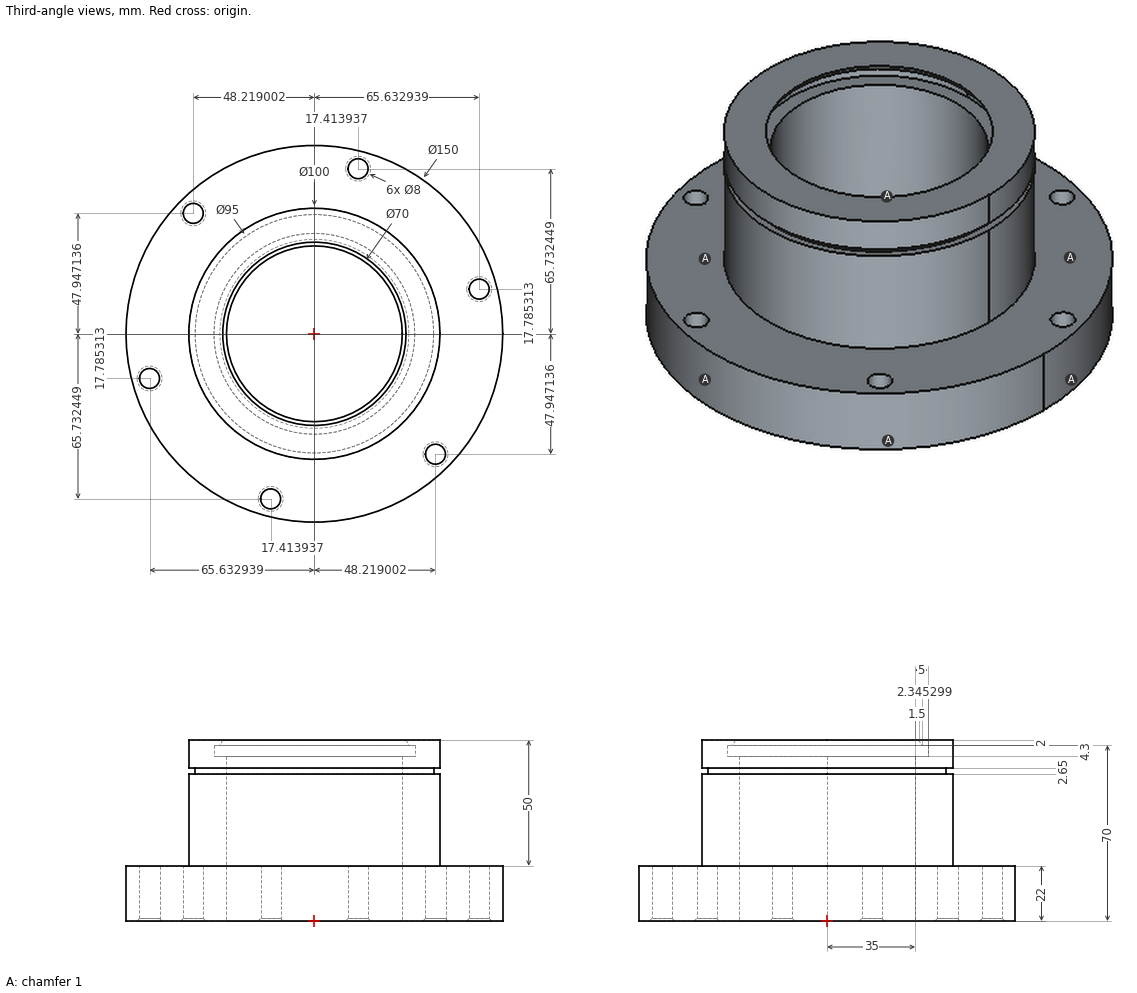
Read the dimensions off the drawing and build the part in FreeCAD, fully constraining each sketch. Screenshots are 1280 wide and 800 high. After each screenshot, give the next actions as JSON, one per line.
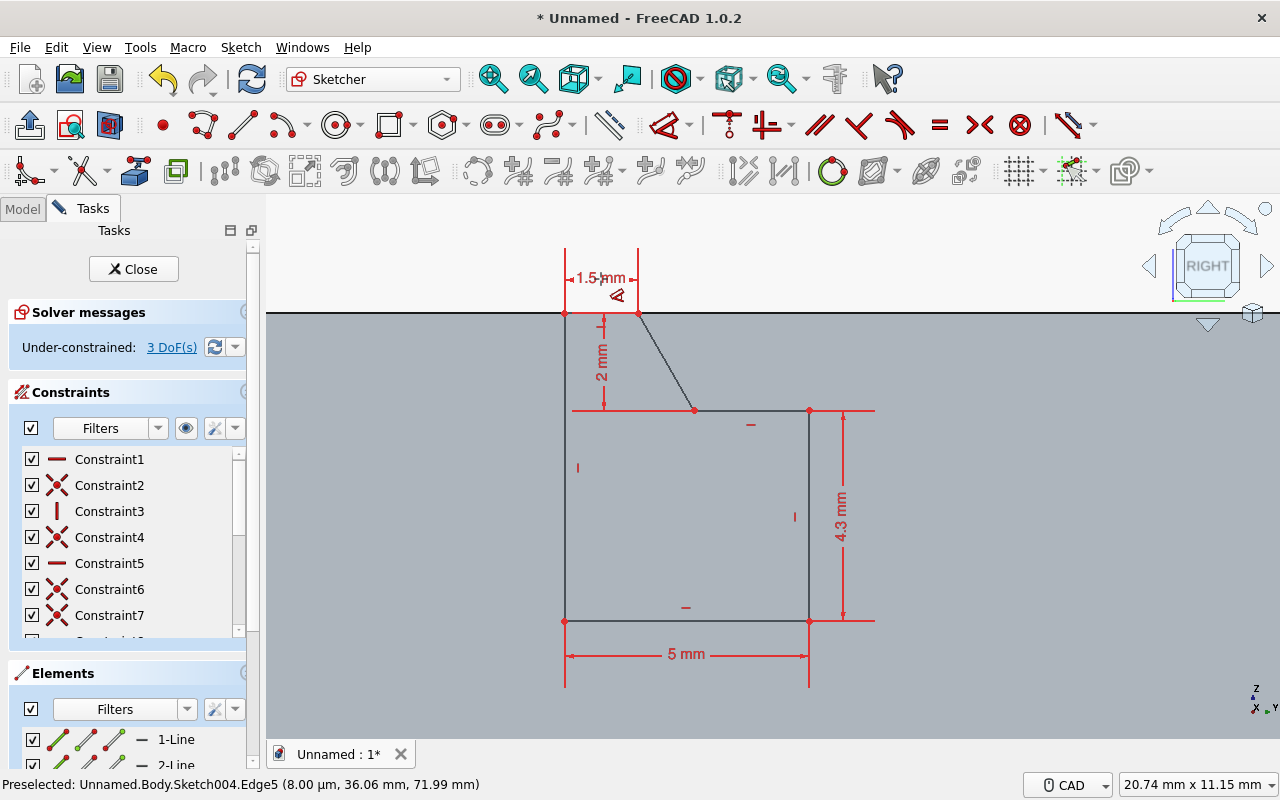
{"action": "left_click", "coordinate": [565, 621]}
{"action": "left_click", "coordinate": [429, 587]}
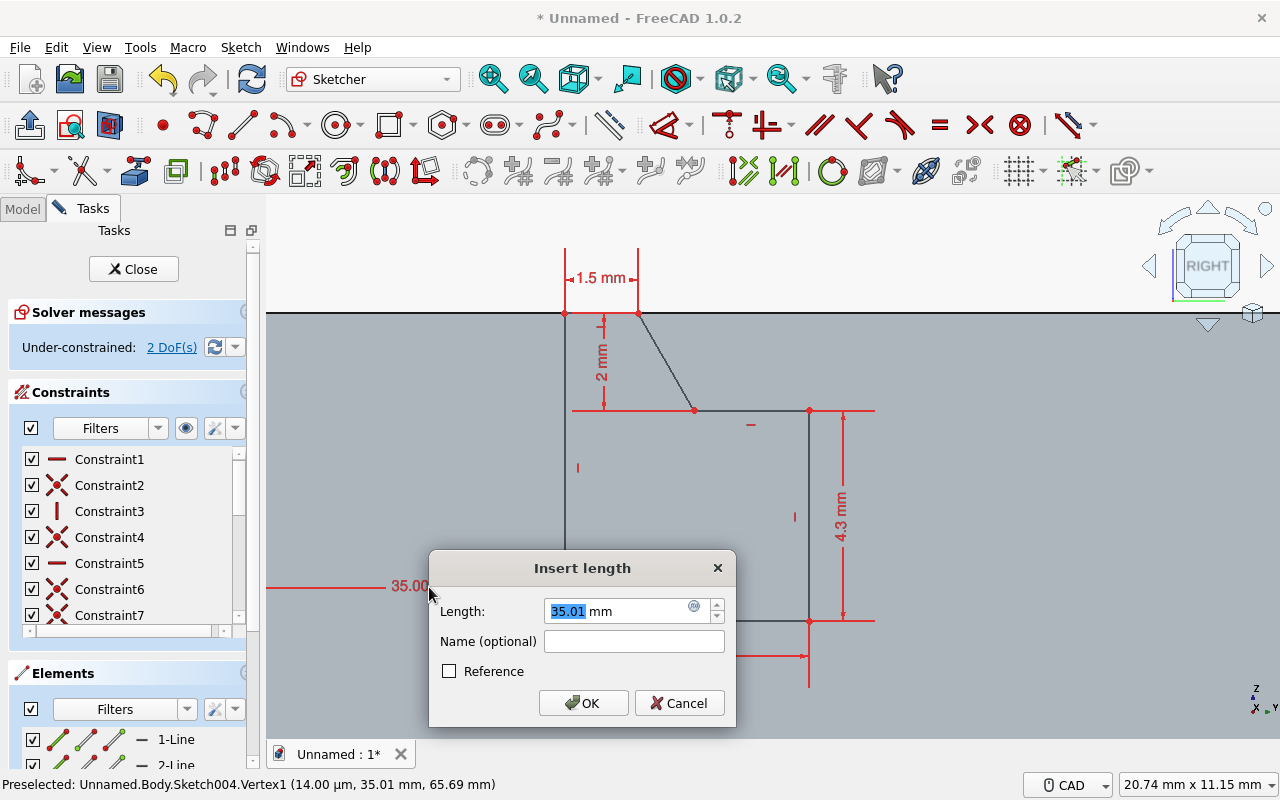
{"action": "type", "text": "35"}
{"action": "key", "text": "Return"}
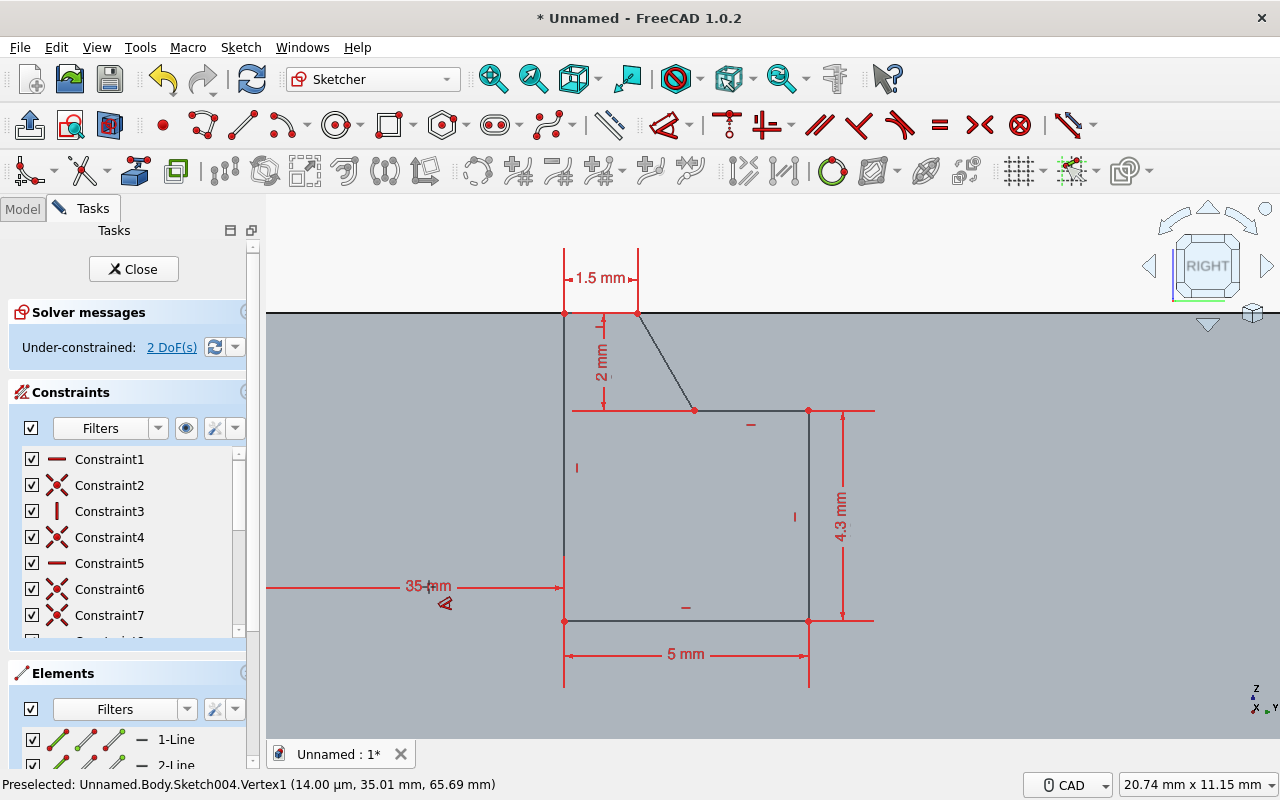
{"action": "left_click", "coordinate": [809, 411]}
{"action": "left_click", "coordinate": [843, 561]}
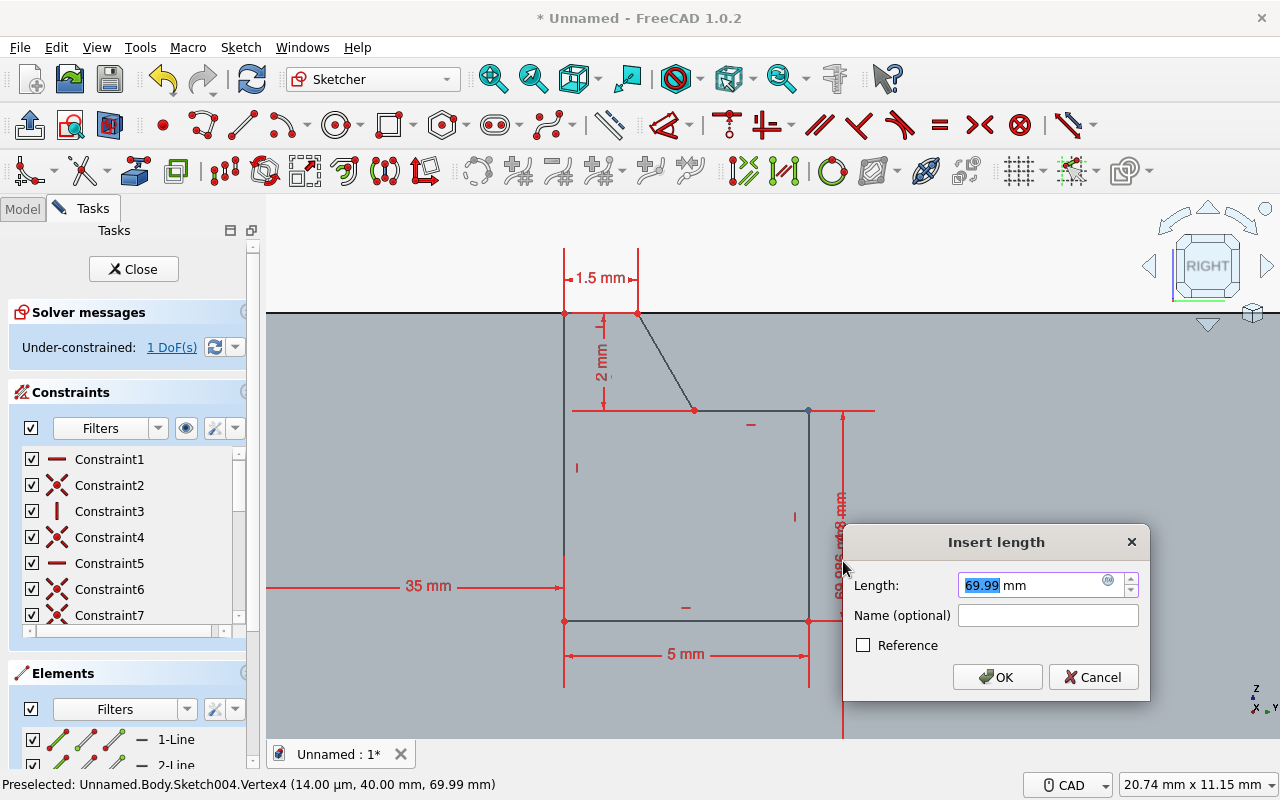
{"action": "type", "text": "70"}
{"action": "key", "text": "Return"}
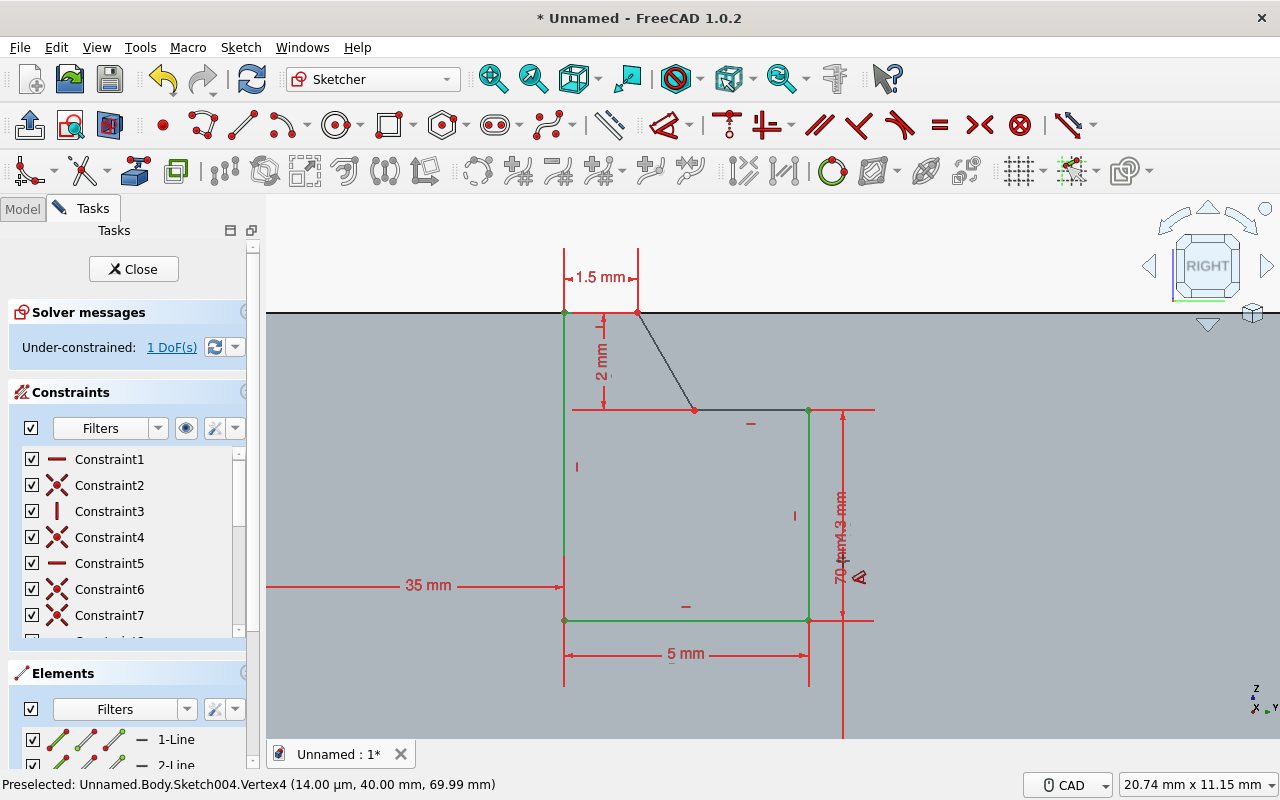
{"action": "left_click", "coordinate": [774, 410]}
{"action": "left_click", "coordinate": [751, 376]}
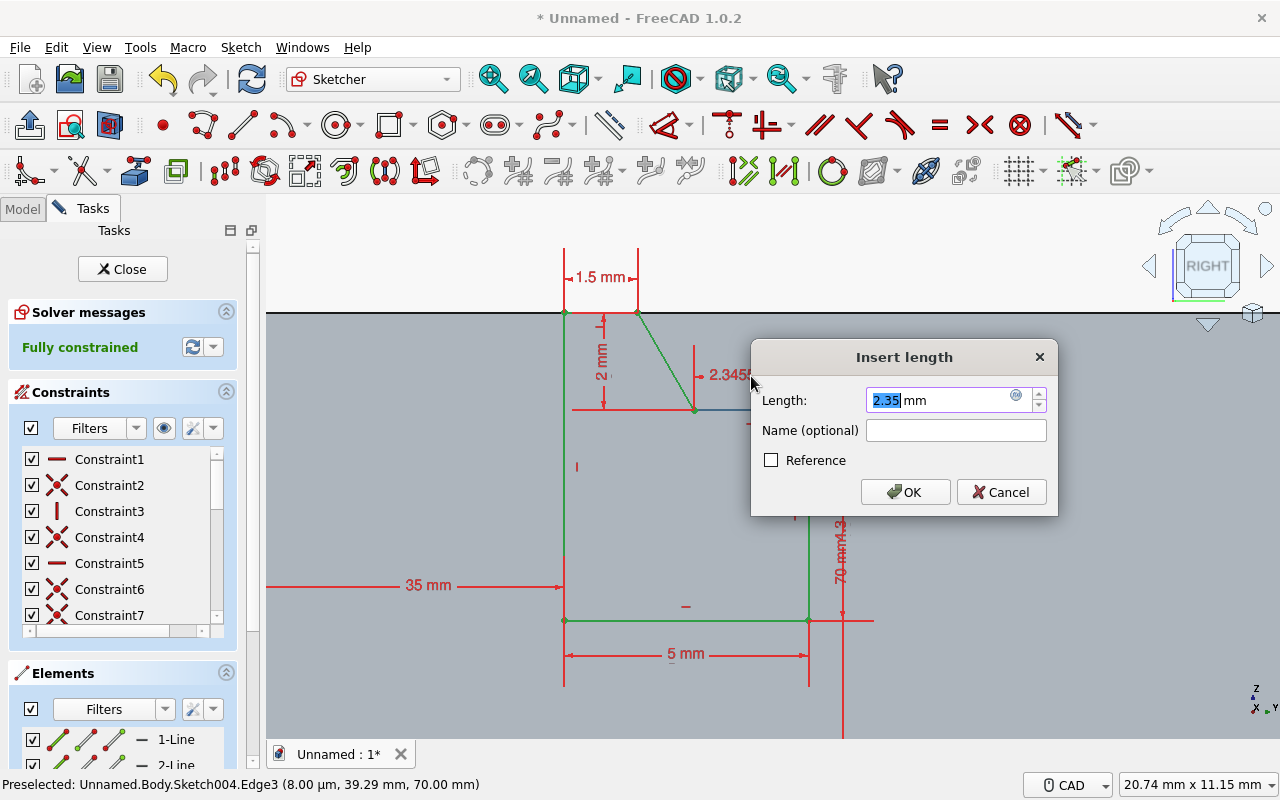
{"action": "type", "text": "2.345299"}
{"action": "key", "text": "Return"}
{"action": "key", "text": "Escape"}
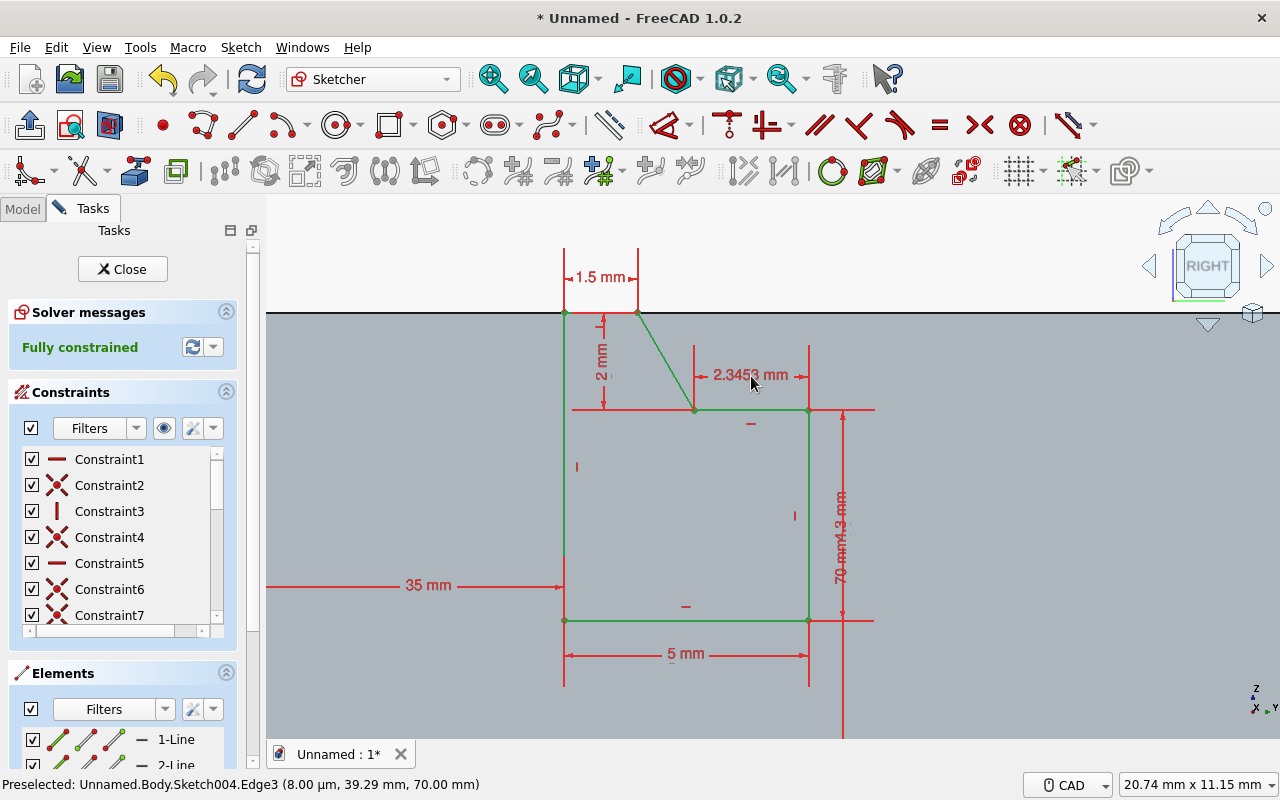
{"action": "left_click", "coordinate": [123, 269]}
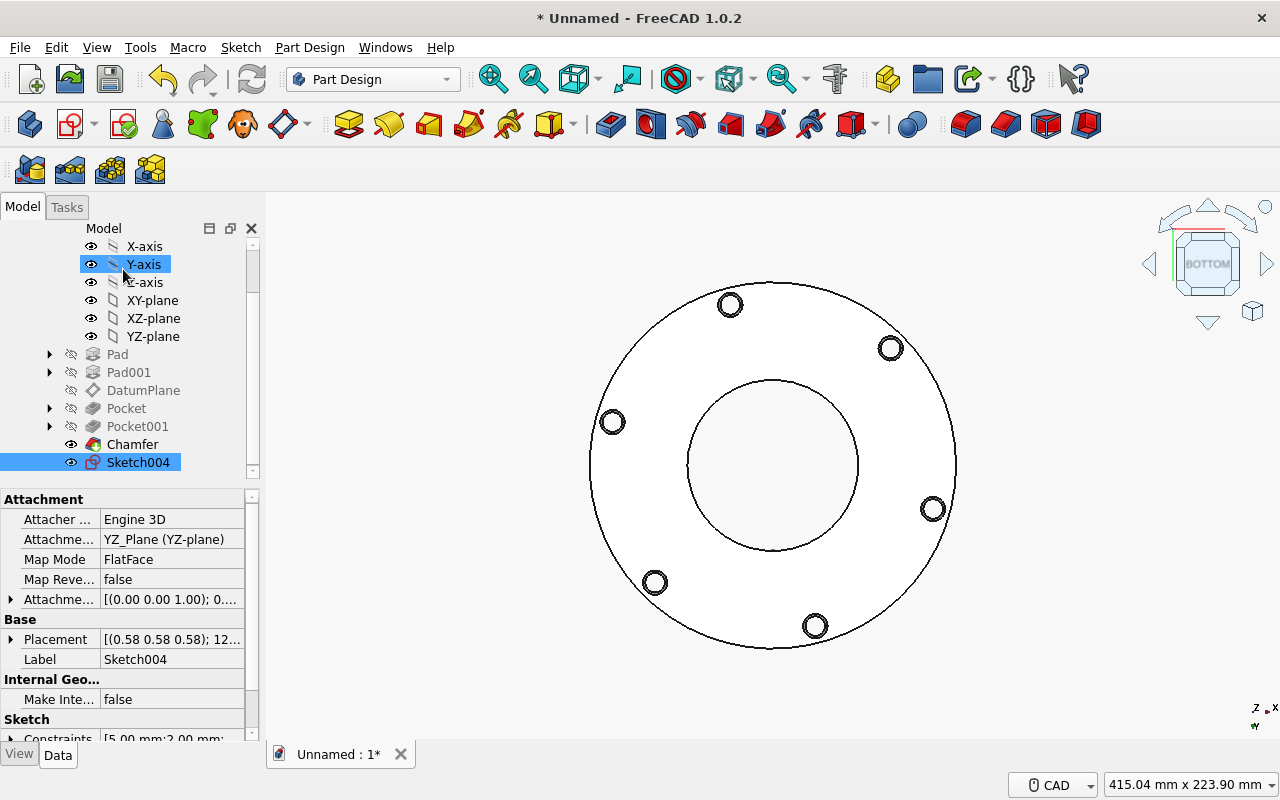
{"action": "left_click", "coordinate": [692, 124]}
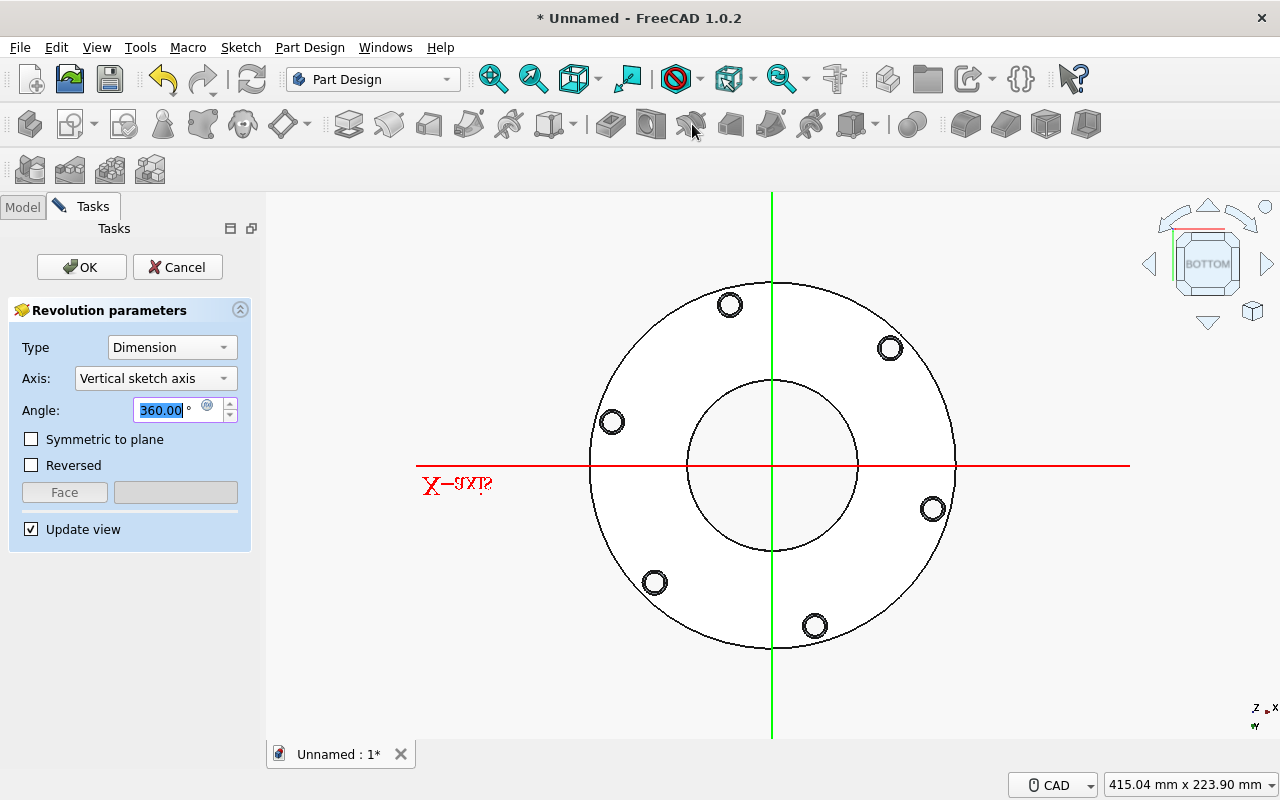
{"action": "left_click", "coordinate": [82, 267]}